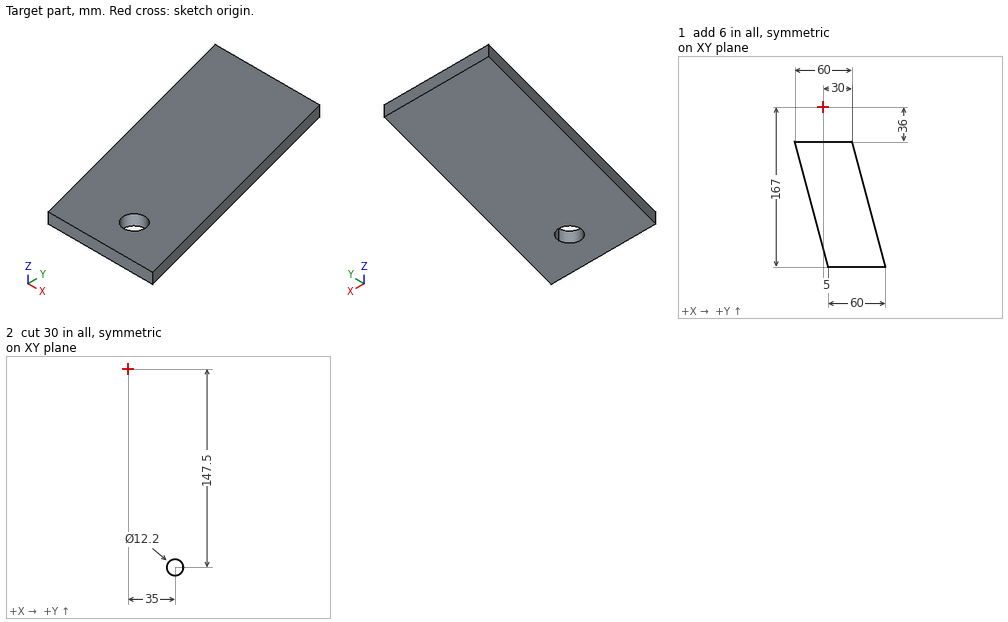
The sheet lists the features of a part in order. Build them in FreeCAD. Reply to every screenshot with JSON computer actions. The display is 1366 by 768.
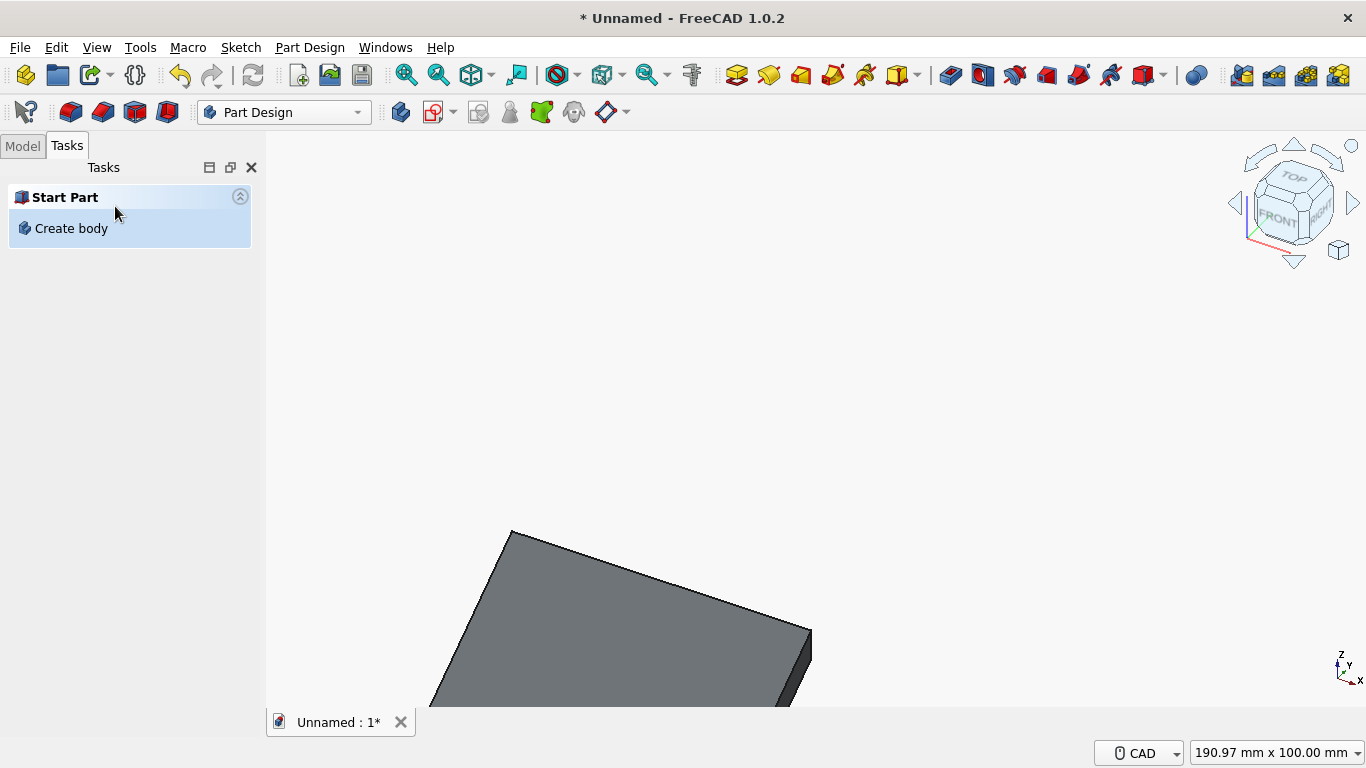
{"action": "left_click", "coordinate": [408, 76]}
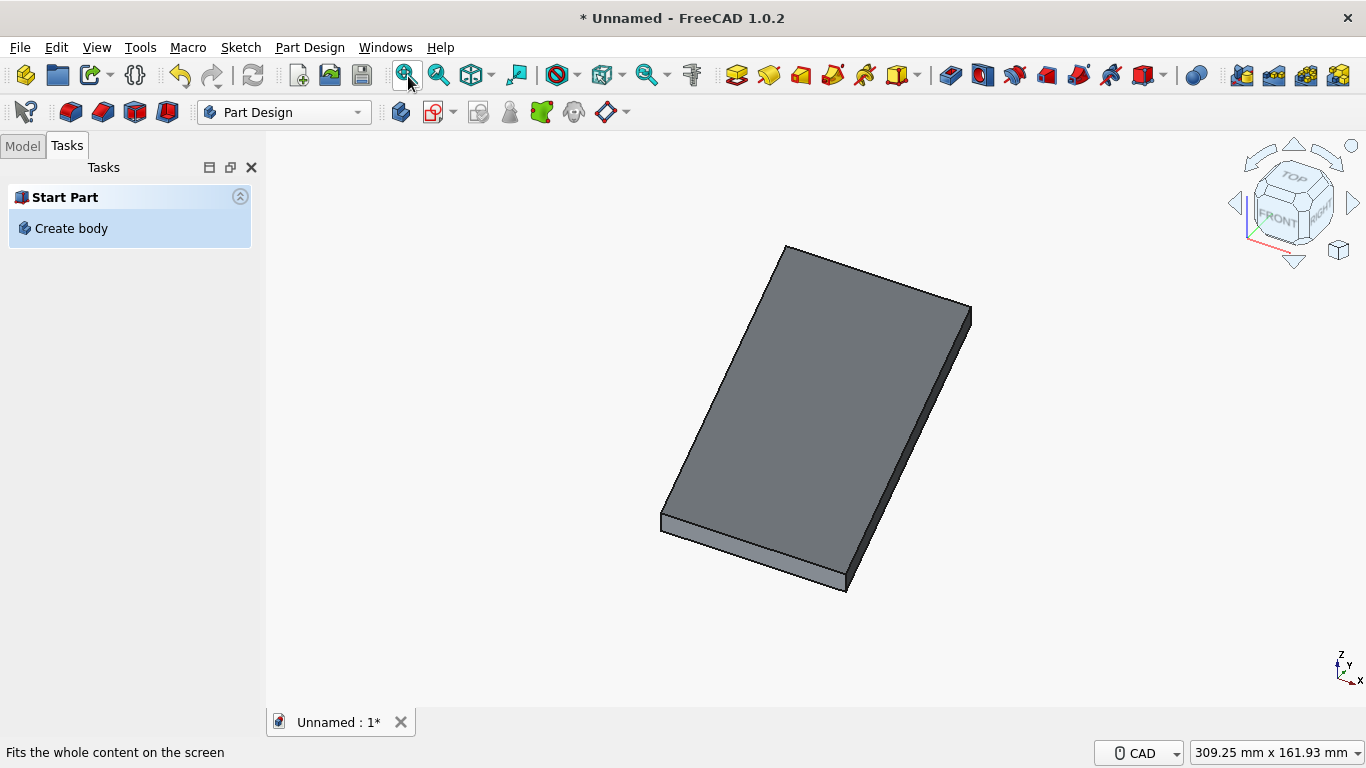
{"action": "left_click", "coordinate": [434, 112]}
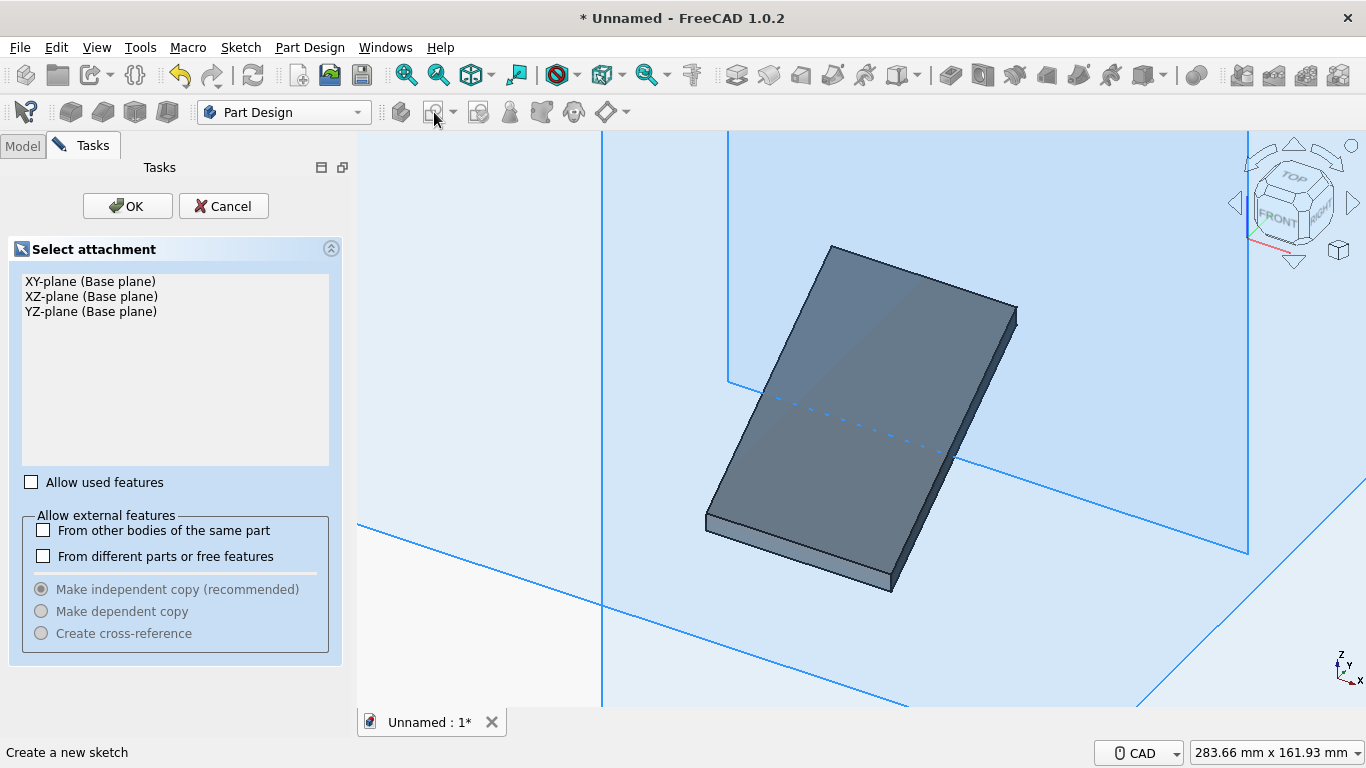
{"action": "left_click", "coordinate": [82, 282]}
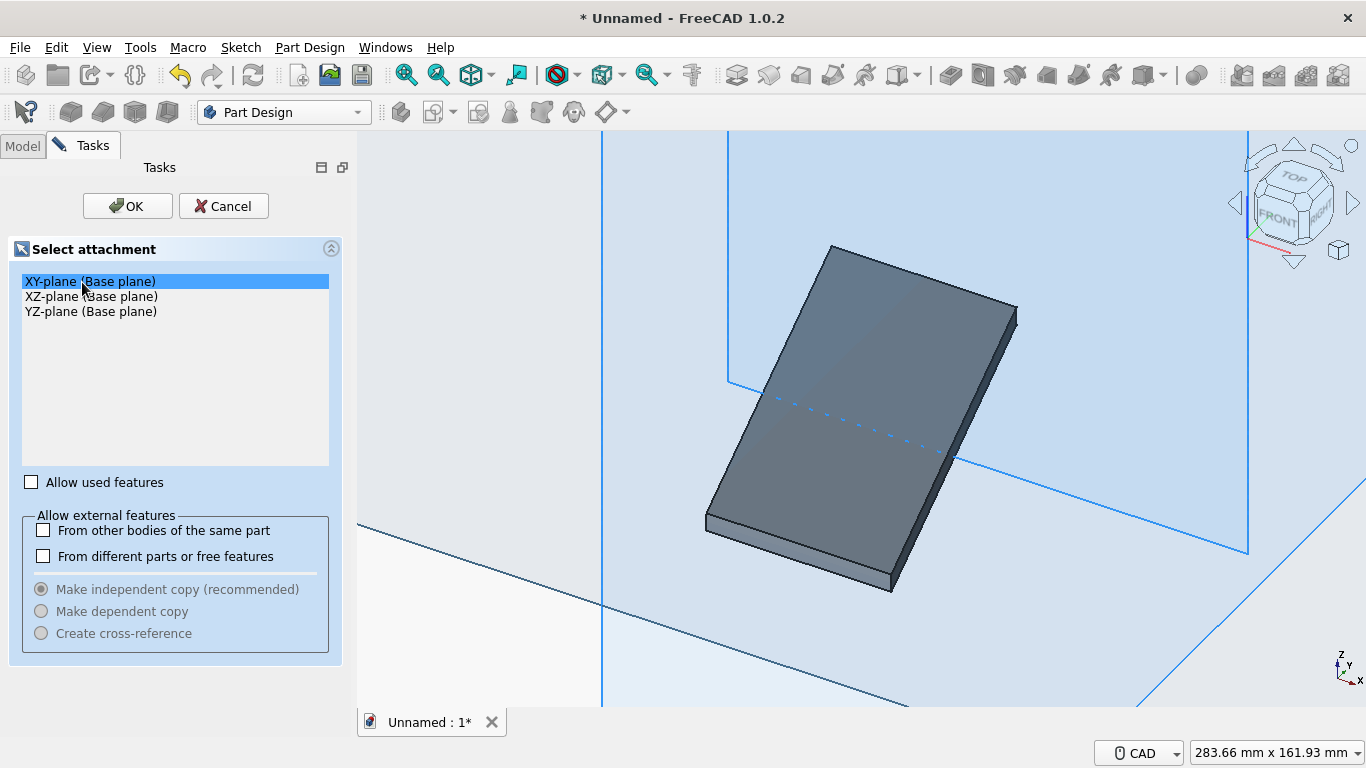
{"action": "left_click", "coordinate": [128, 206]}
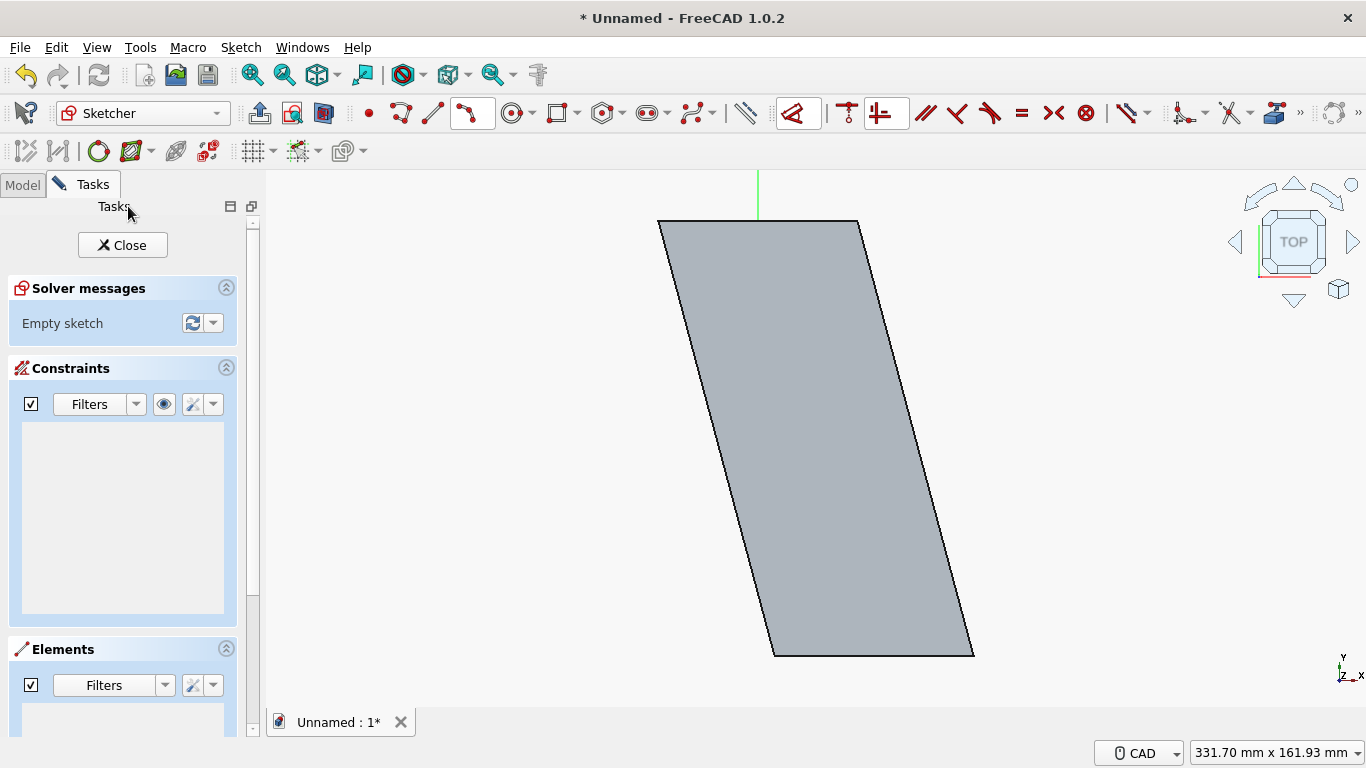
{"action": "left_click", "coordinate": [324, 114]}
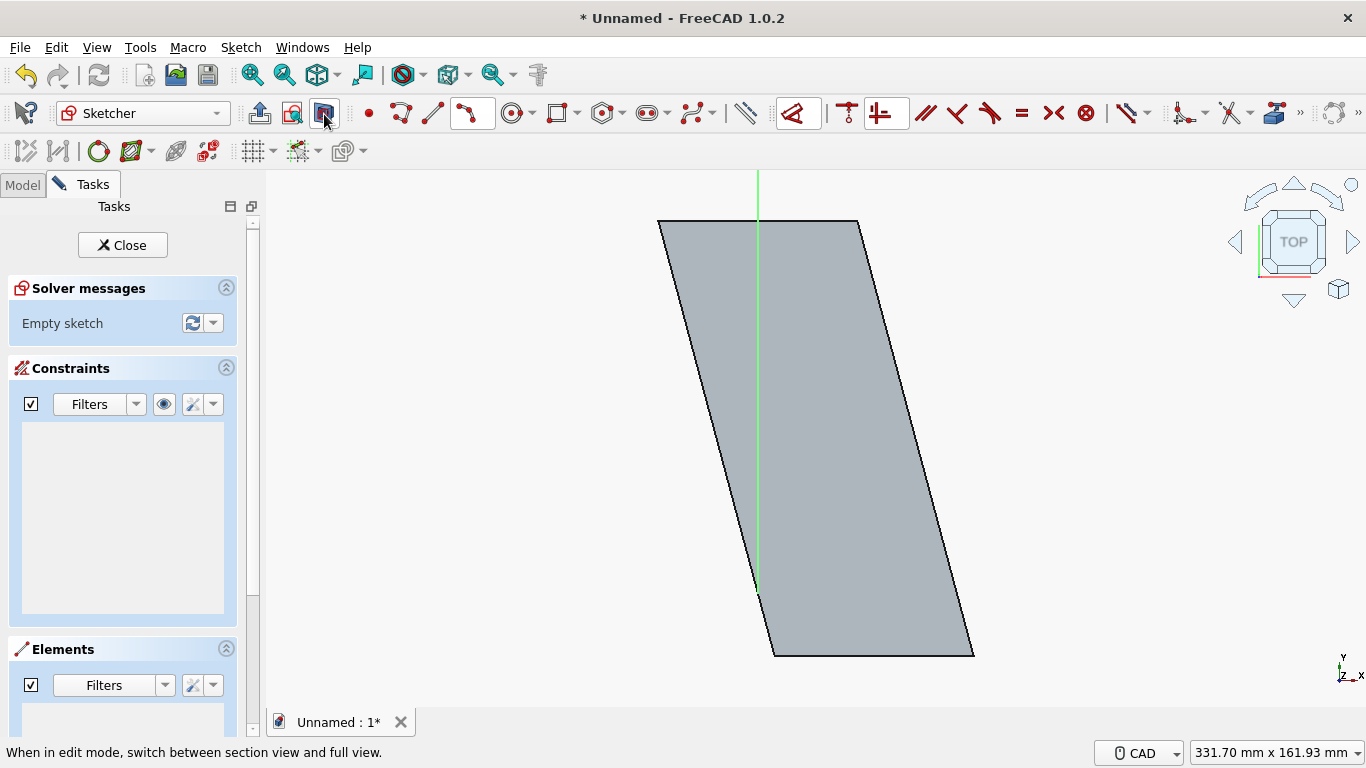
{"action": "scroll", "coordinate": [890, 610], "scroll_direction": "up", "scroll_amount": 11}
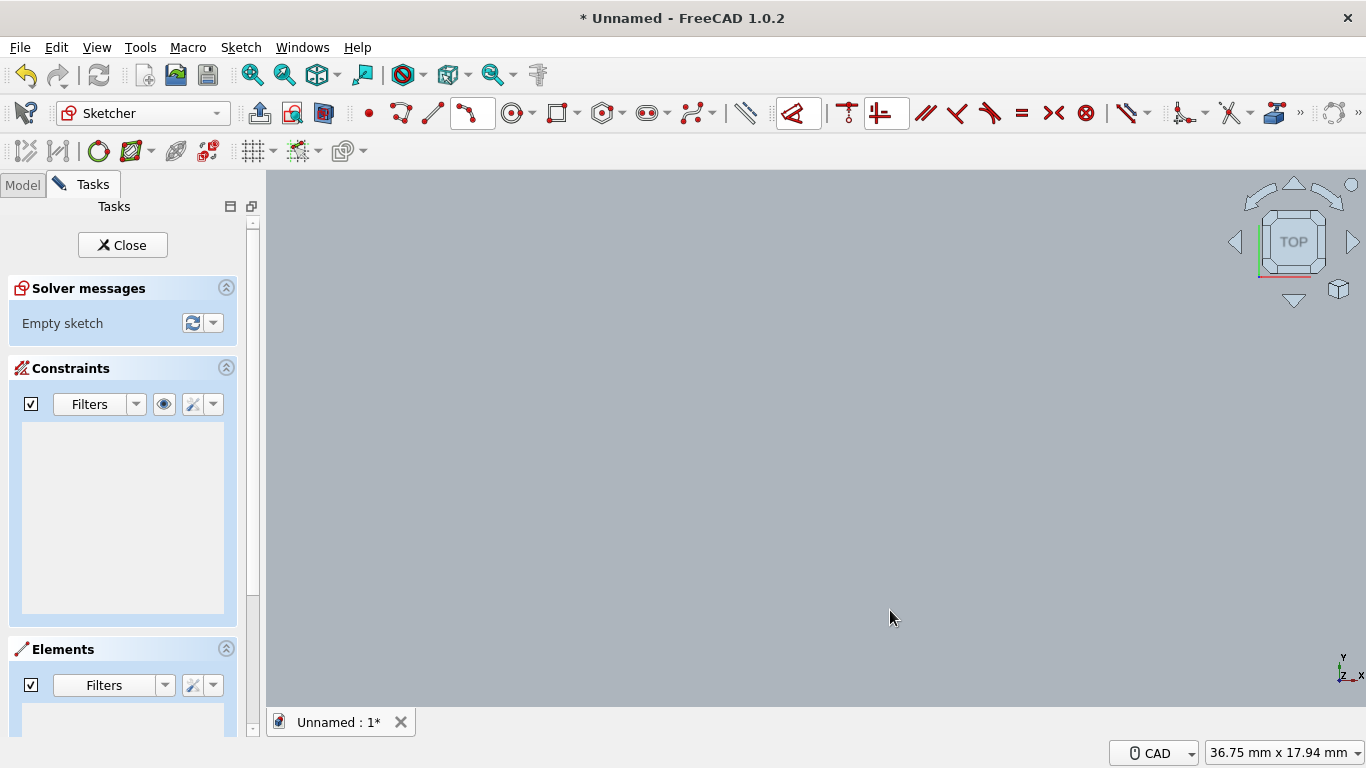
{"action": "left_click", "coordinate": [512, 114]}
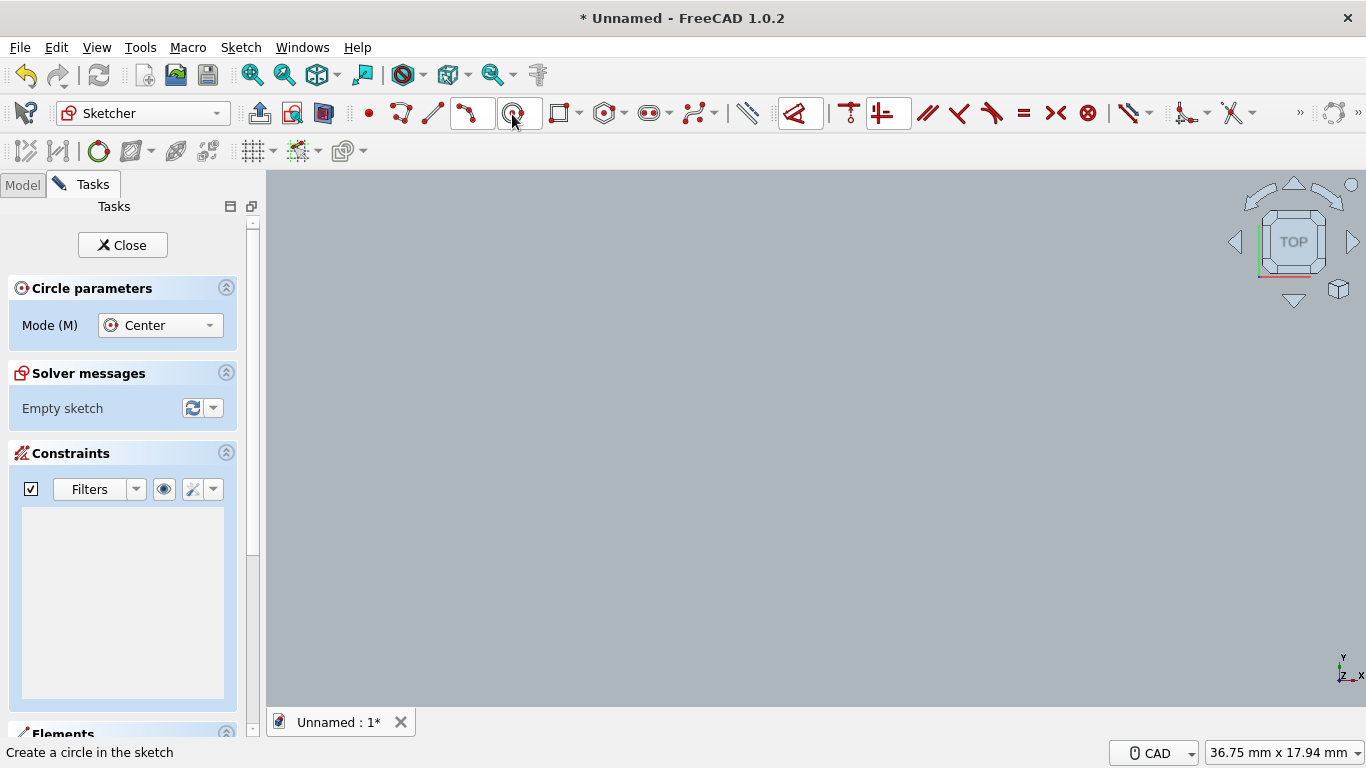
{"action": "left_click", "coordinate": [741, 432]}
{"action": "mouse_move", "coordinate": [870, 303]}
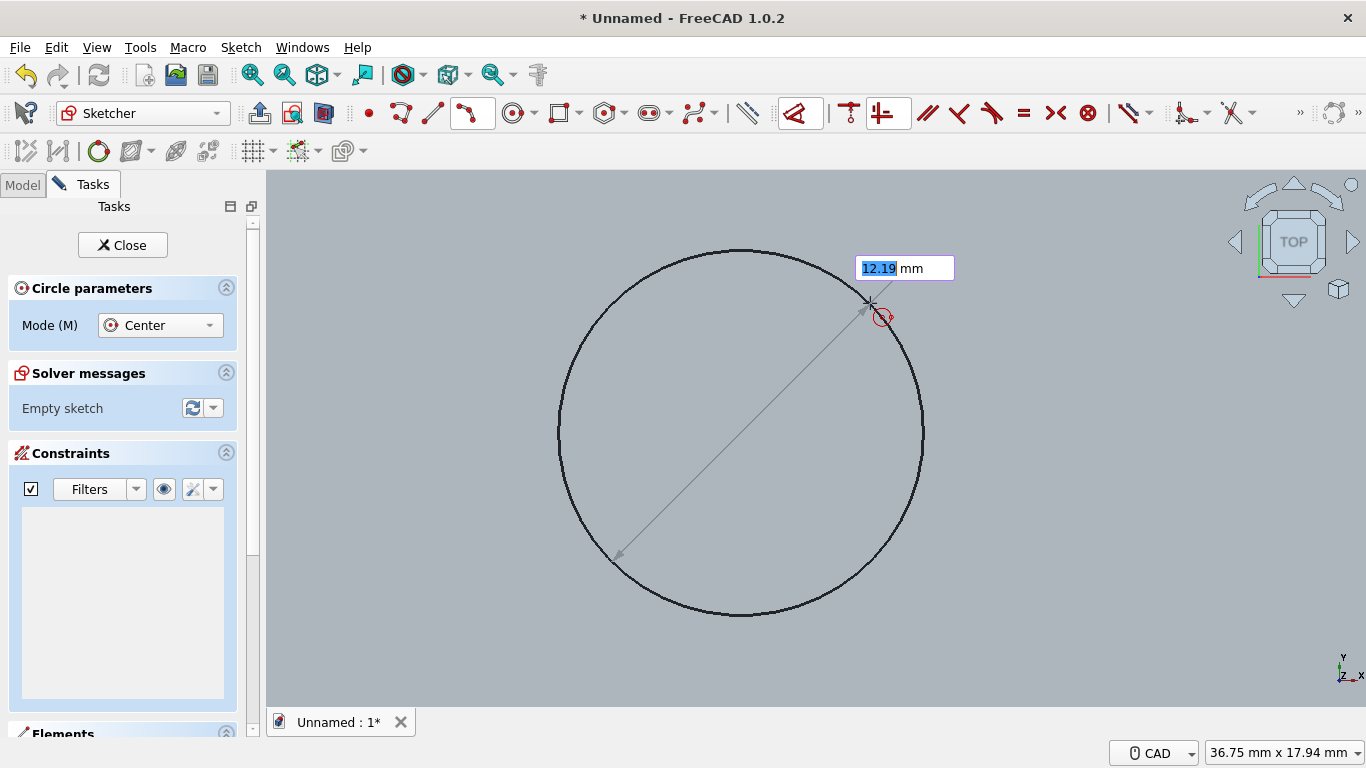
{"action": "type", "text": "12.2"}
{"action": "key", "text": "Return"}
{"action": "key", "text": "Escape"}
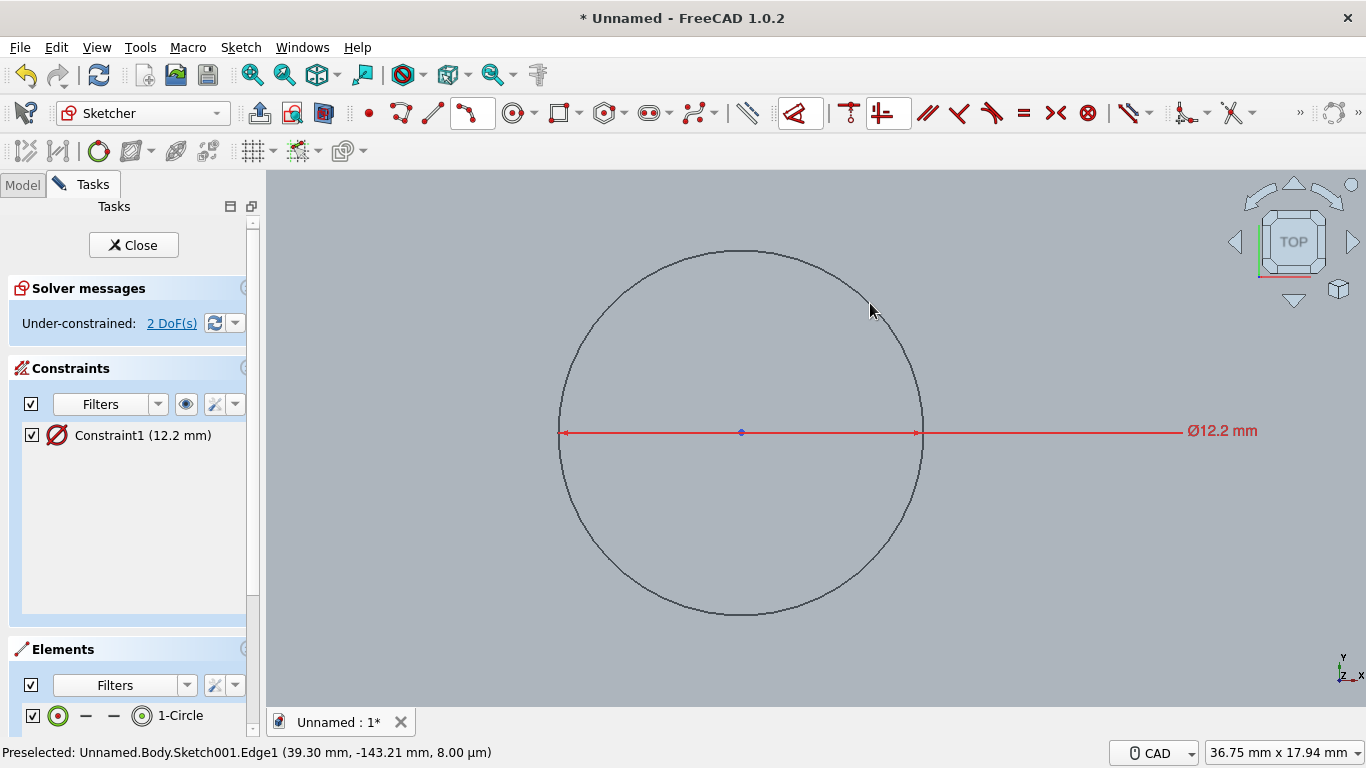
{"action": "left_click", "coordinate": [741, 433]}